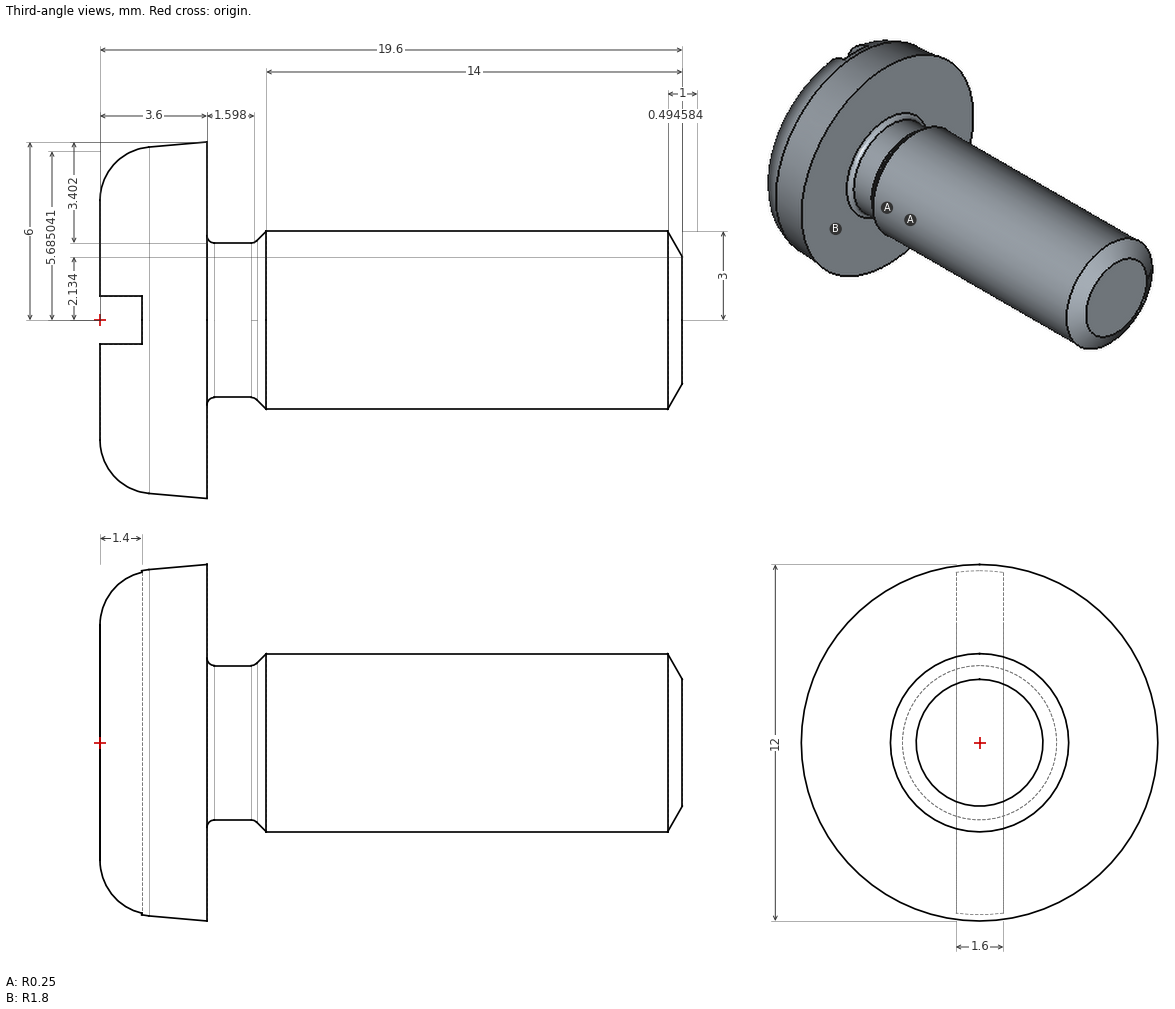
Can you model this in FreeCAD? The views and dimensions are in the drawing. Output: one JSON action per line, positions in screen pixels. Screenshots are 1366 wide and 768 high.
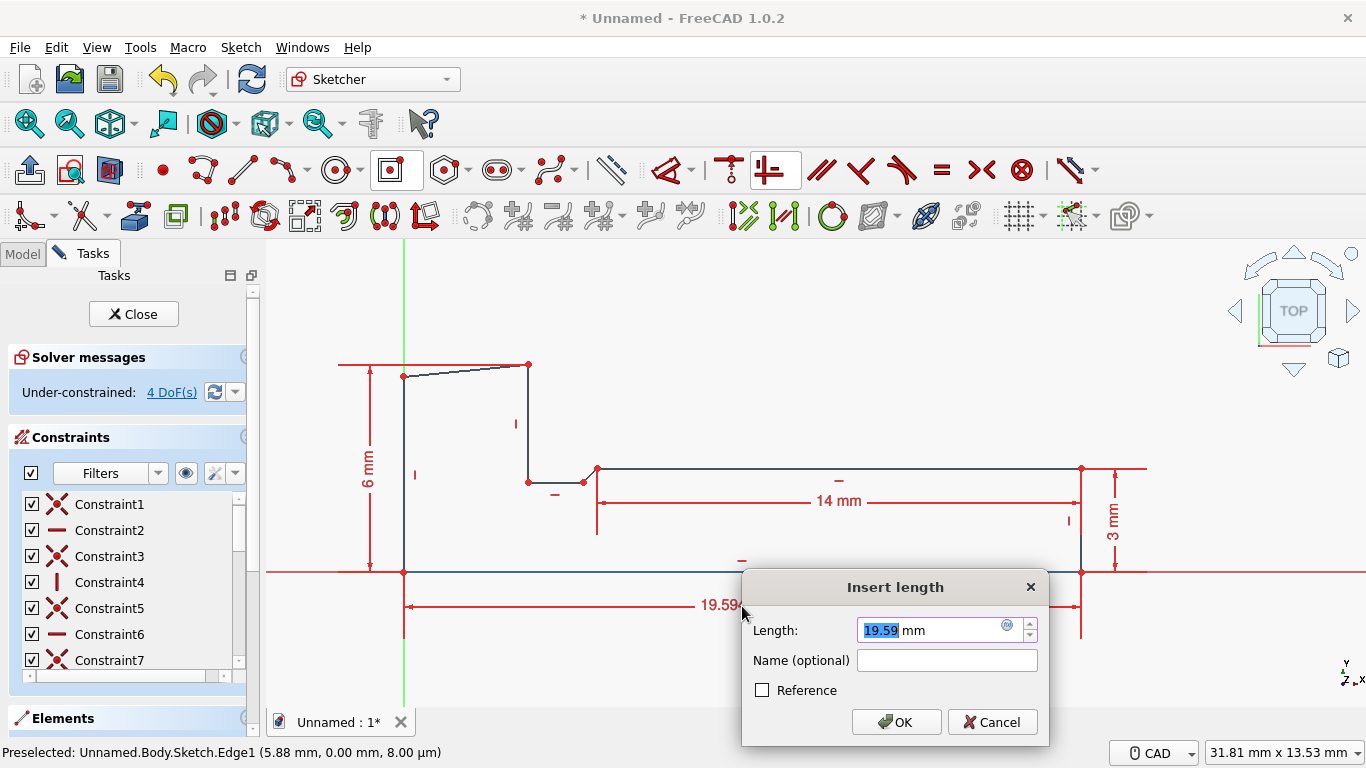
{"action": "type", "text": "19.6"}
{"action": "key", "text": "Return"}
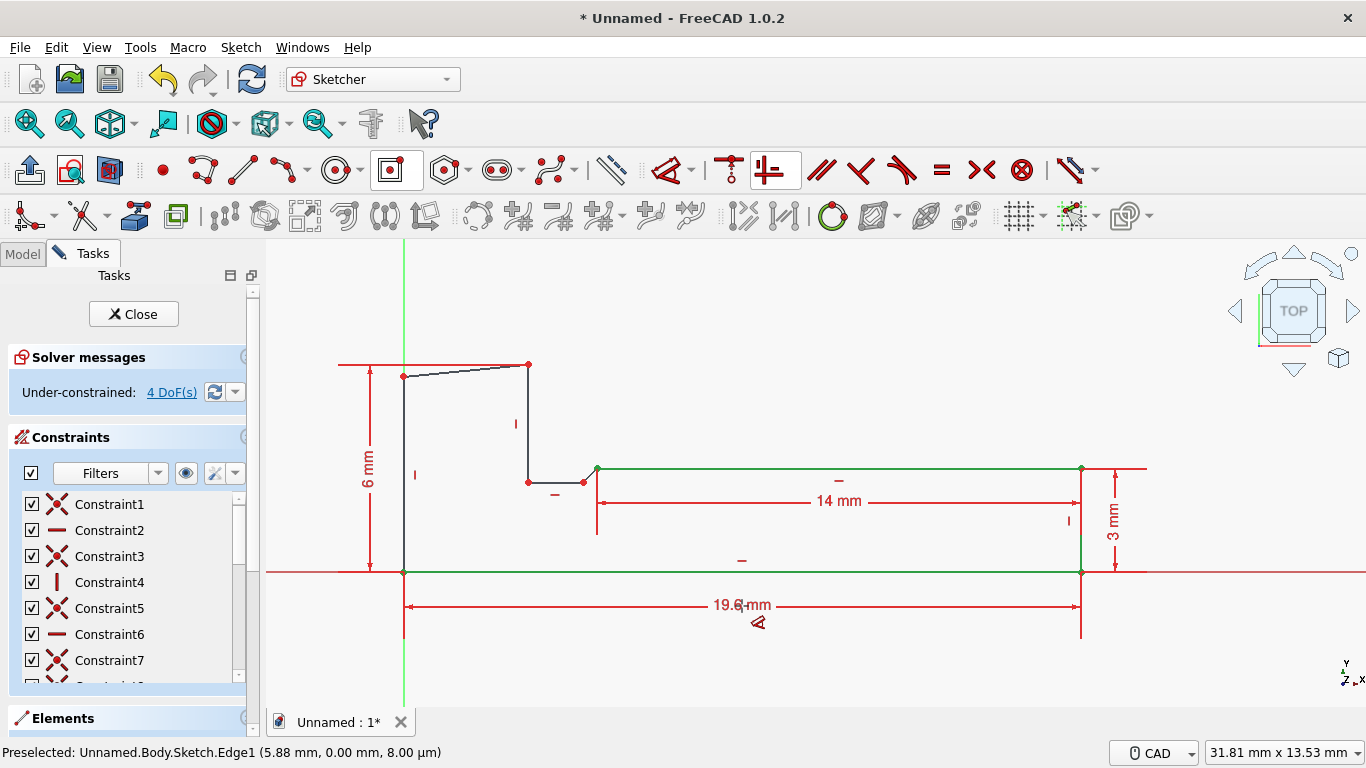
{"action": "left_click", "coordinate": [528, 483]}
{"action": "left_click", "coordinate": [466, 606]}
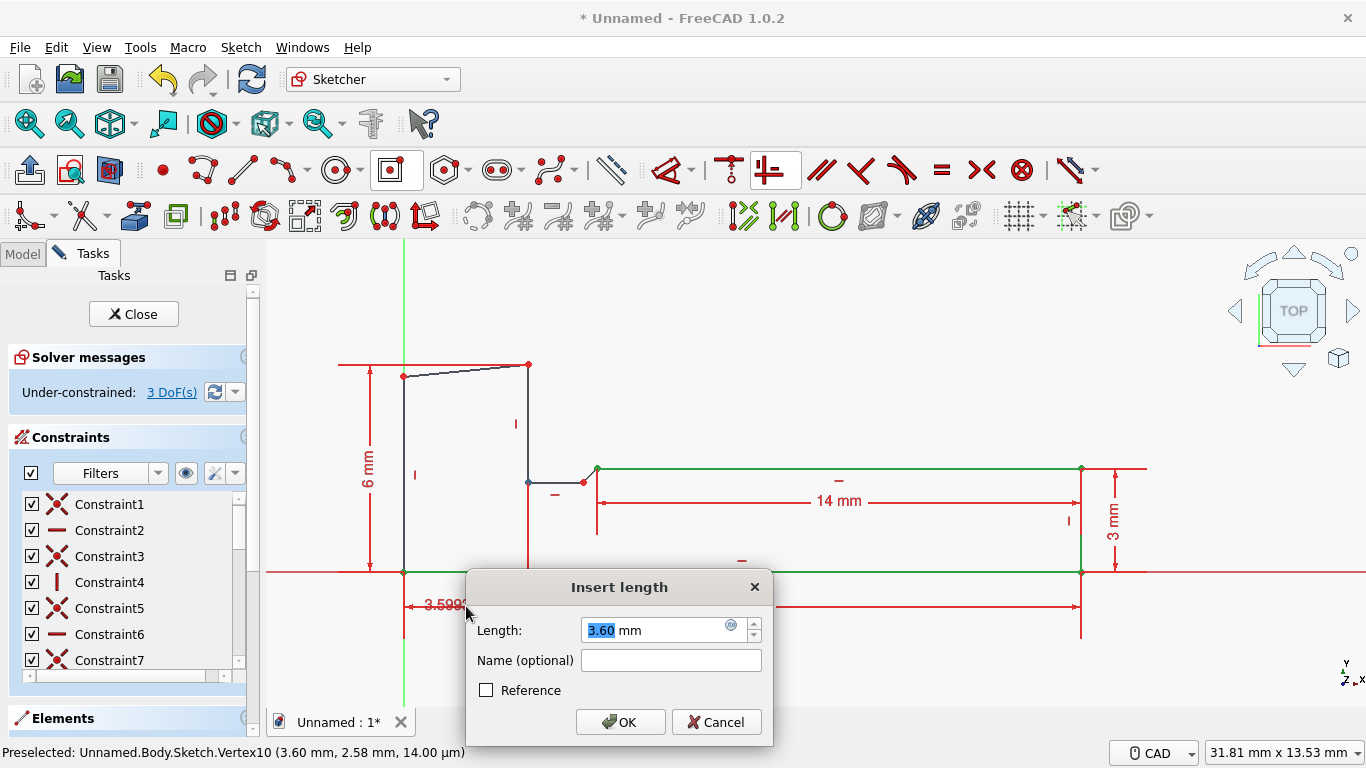
{"action": "type", "text": "3.6"}
{"action": "key", "text": "Return"}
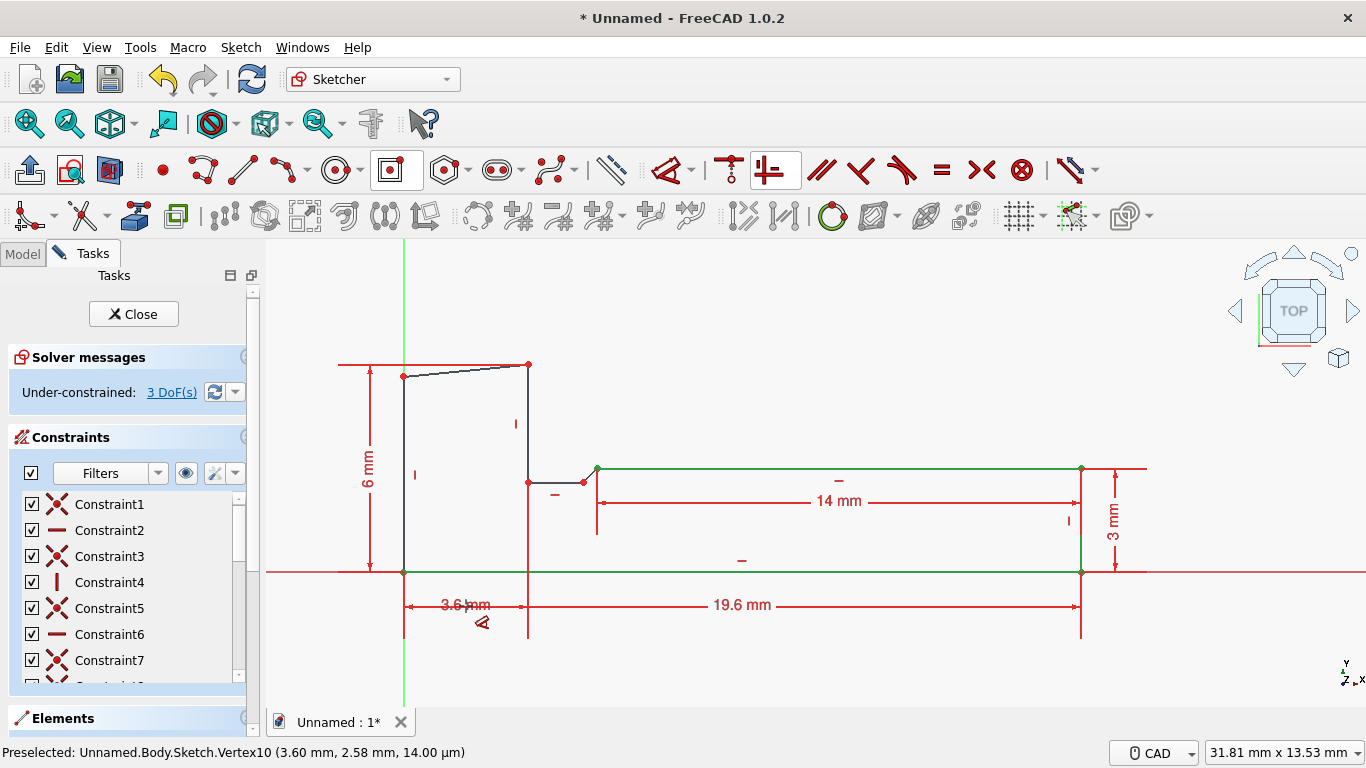
{"action": "left_click", "coordinate": [567, 483]}
{"action": "left_click", "coordinate": [556, 517]}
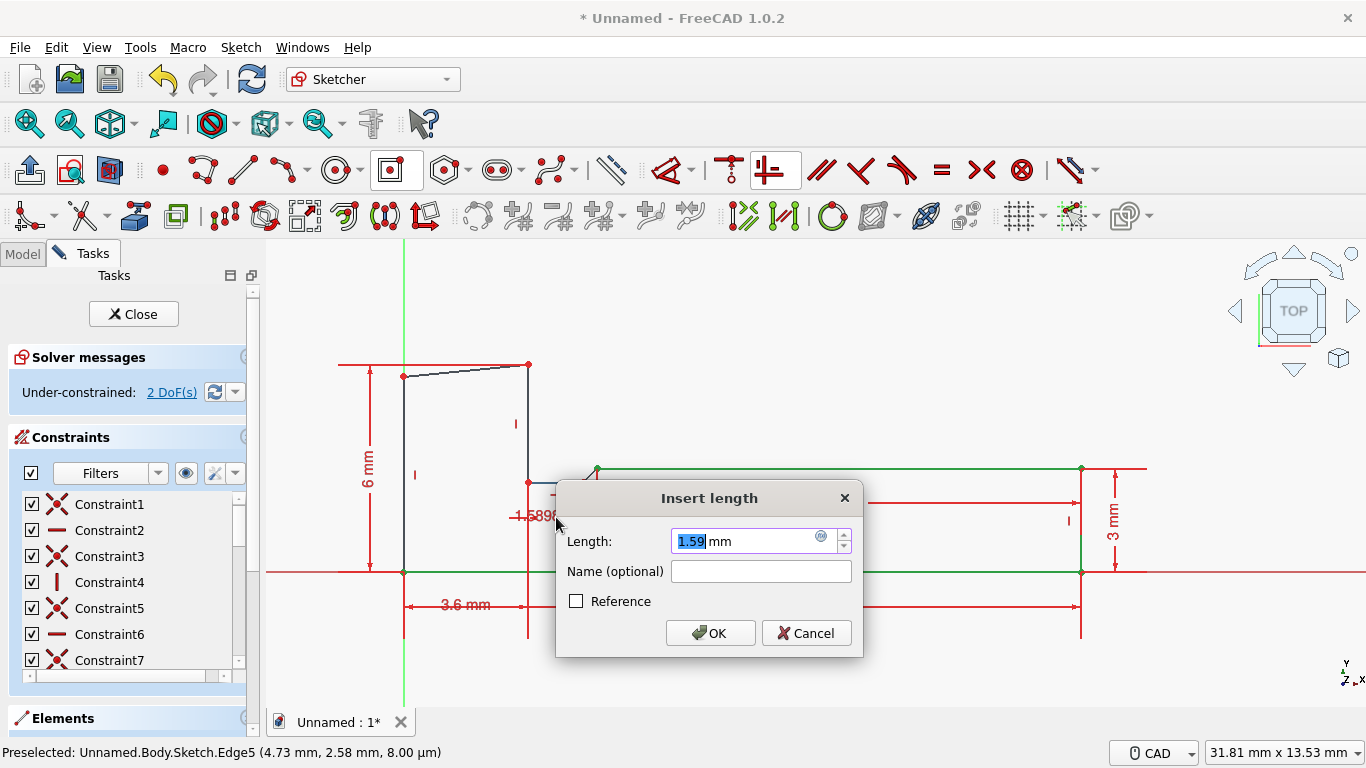
{"action": "type", "text": "1.598"}
{"action": "key", "text": "Return"}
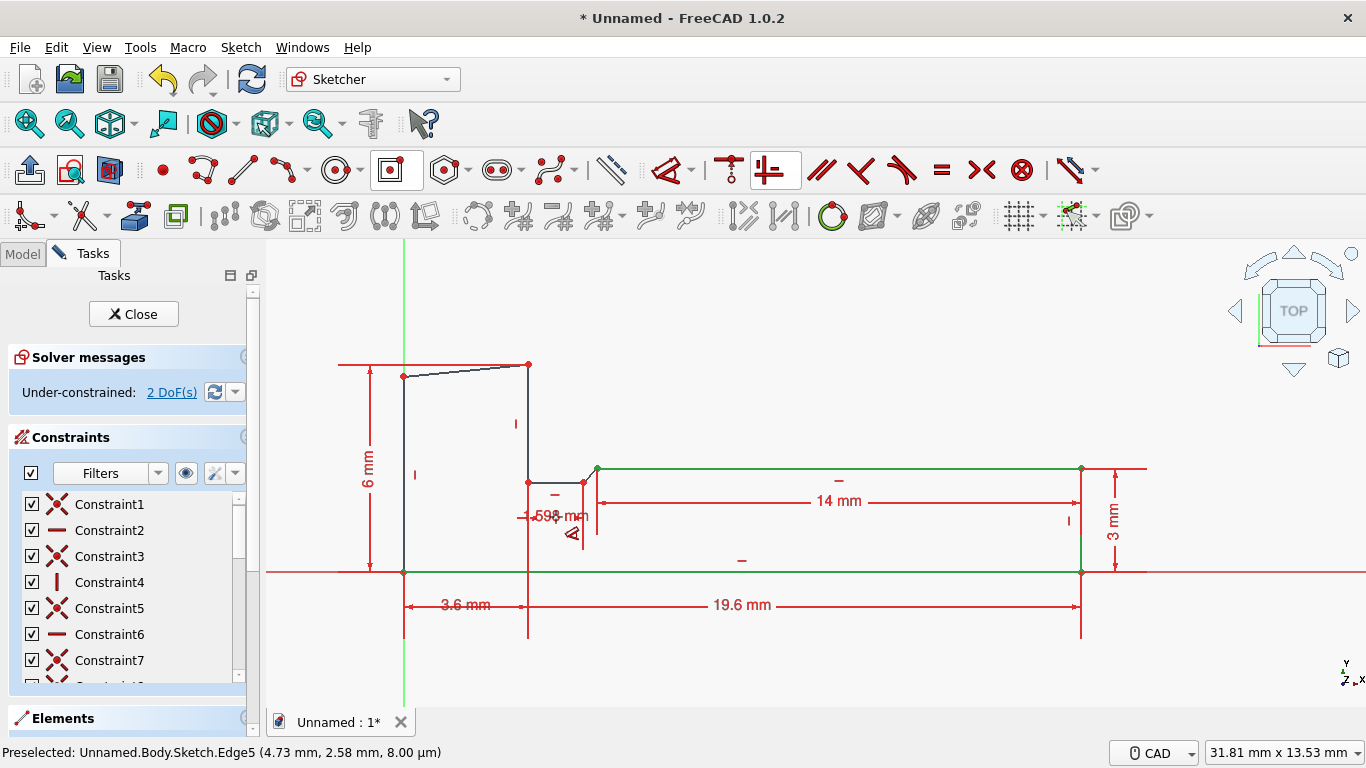
{"action": "left_click", "coordinate": [528, 448]}
{"action": "left_click", "coordinate": [494, 424]}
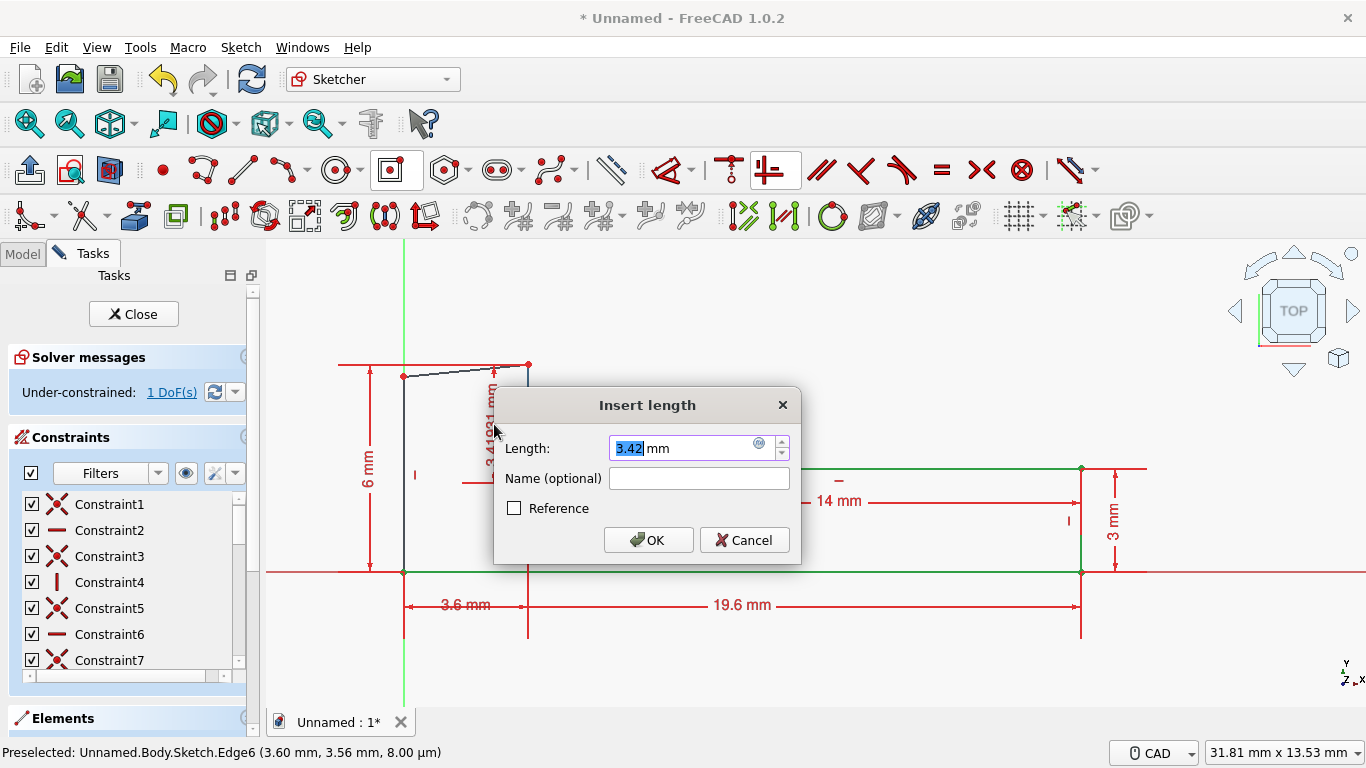
{"action": "type", "text": "3.402"}
{"action": "key", "text": "Return"}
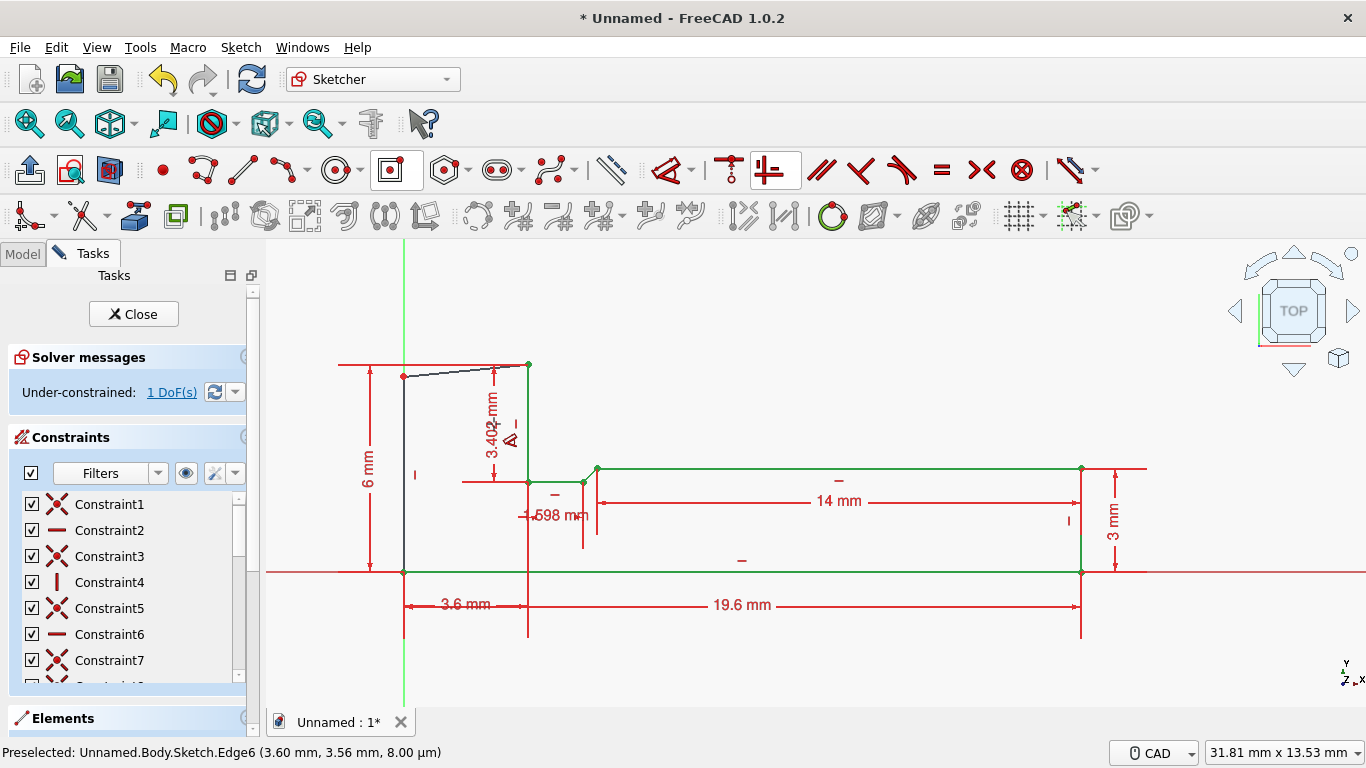
{"action": "left_click", "coordinate": [404, 436]}
{"action": "left_click", "coordinate": [370, 430]}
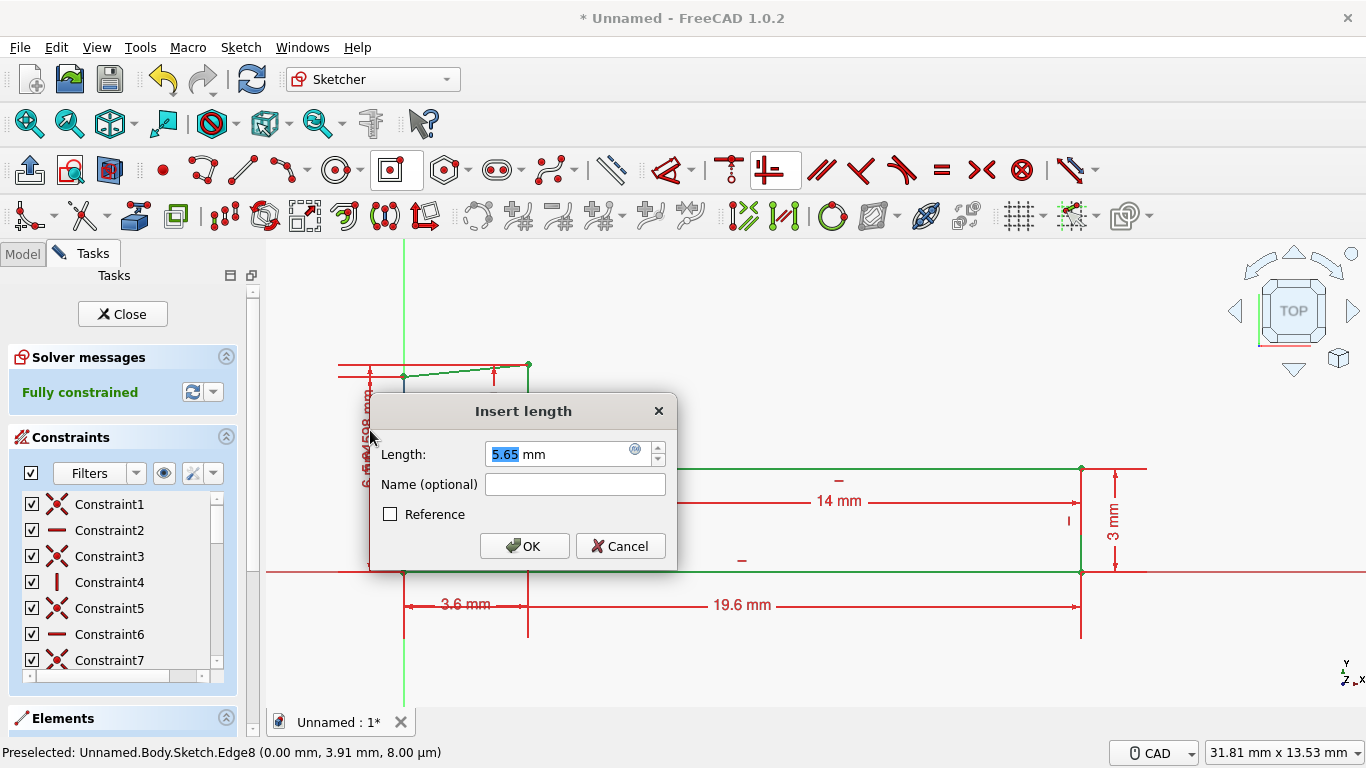
{"action": "type", "text": "5.685041"}
{"action": "key", "text": "Return"}
{"action": "key", "text": "Escape"}